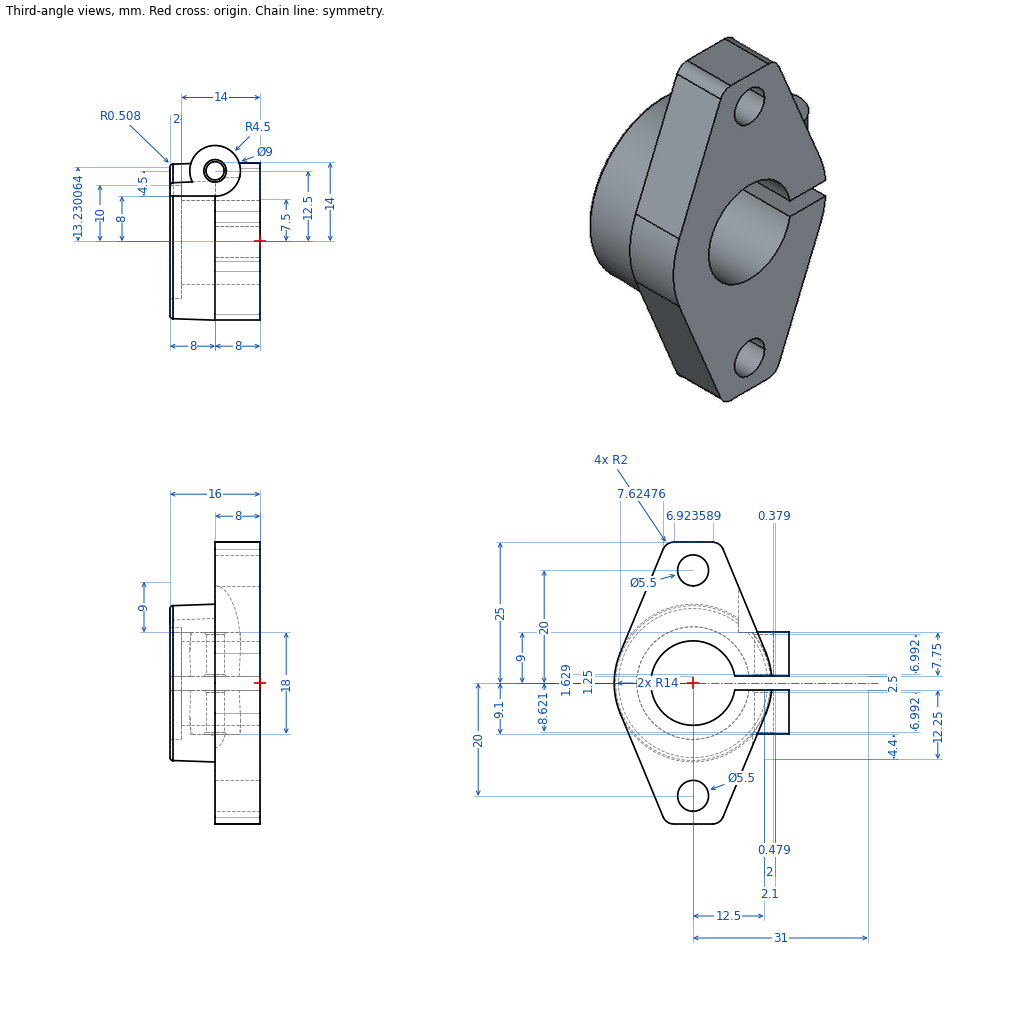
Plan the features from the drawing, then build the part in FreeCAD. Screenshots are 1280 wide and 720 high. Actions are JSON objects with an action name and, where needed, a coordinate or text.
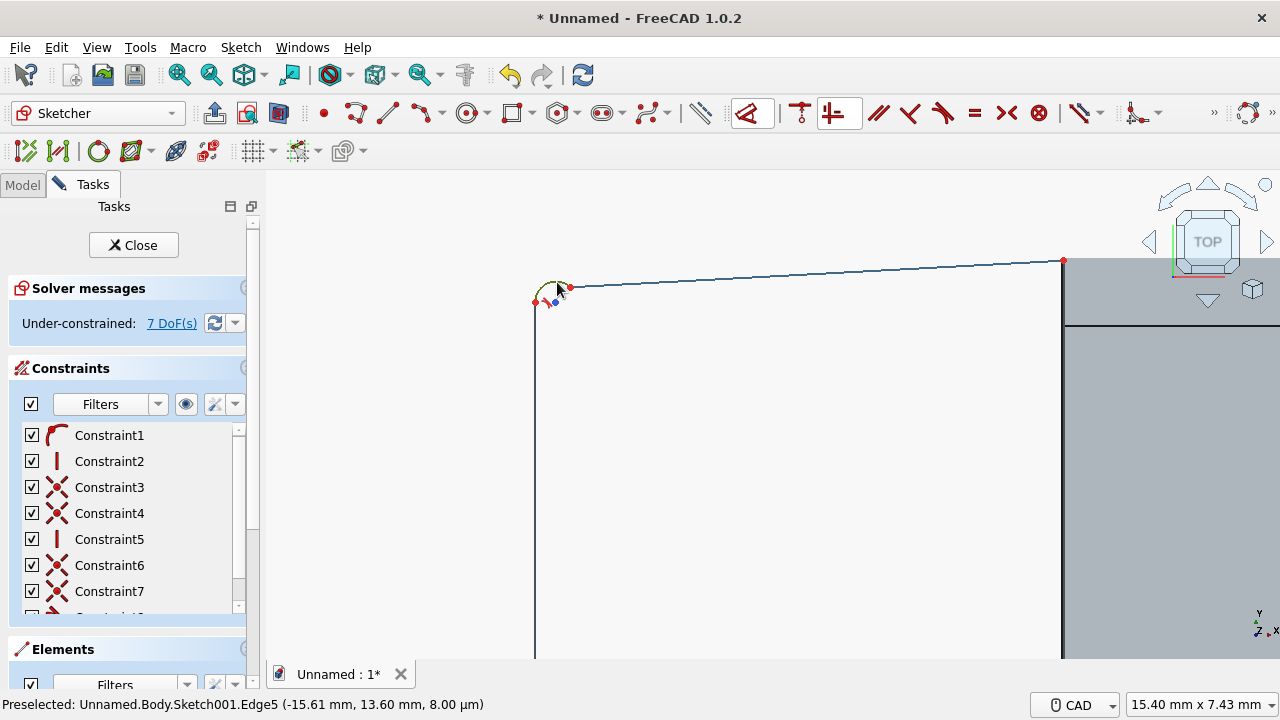
{"action": "left_click", "coordinate": [944, 114]}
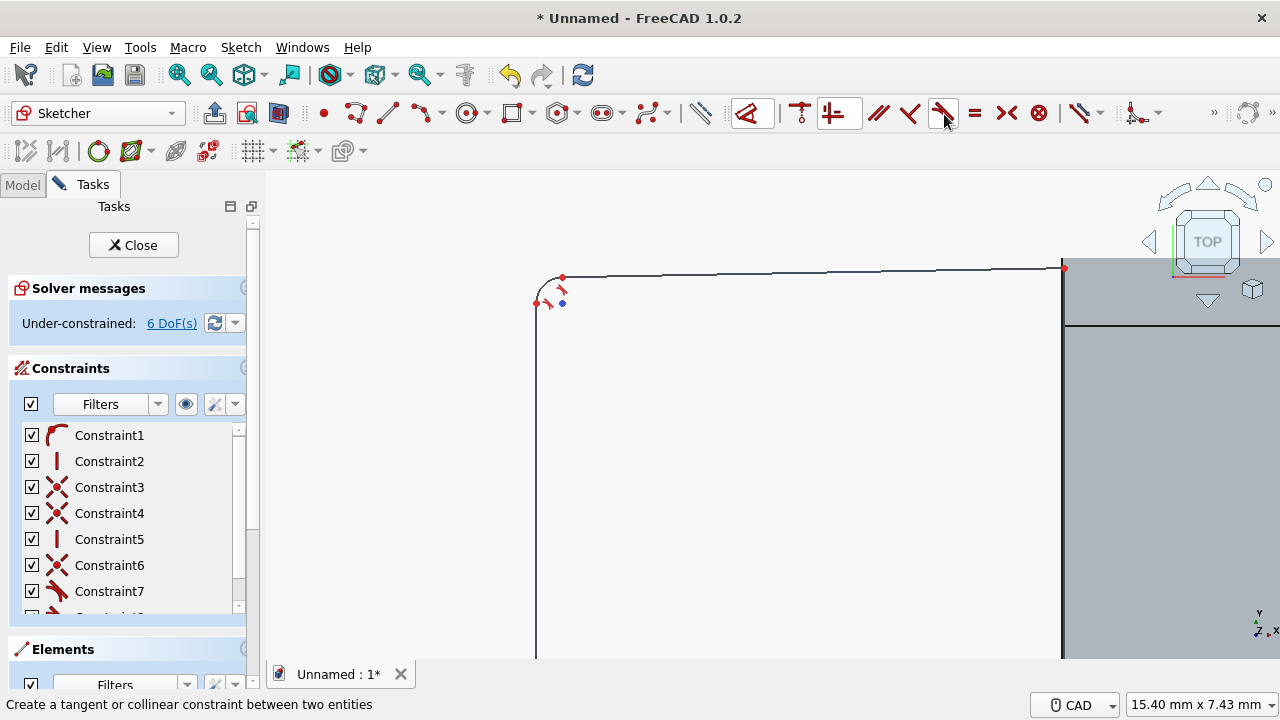
{"action": "scroll", "coordinate": [550, 284], "scroll_direction": "down", "scroll_amount": 6}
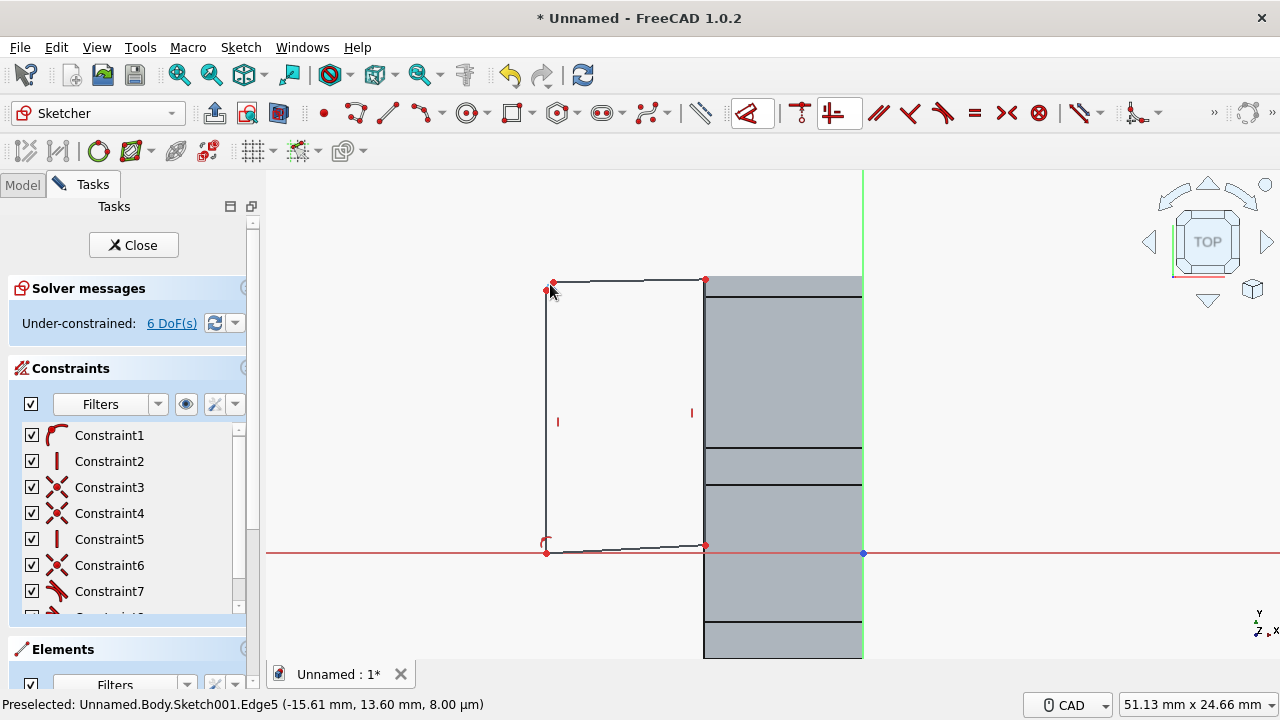
{"action": "scroll", "coordinate": [657, 548], "scroll_direction": "up", "scroll_amount": 5}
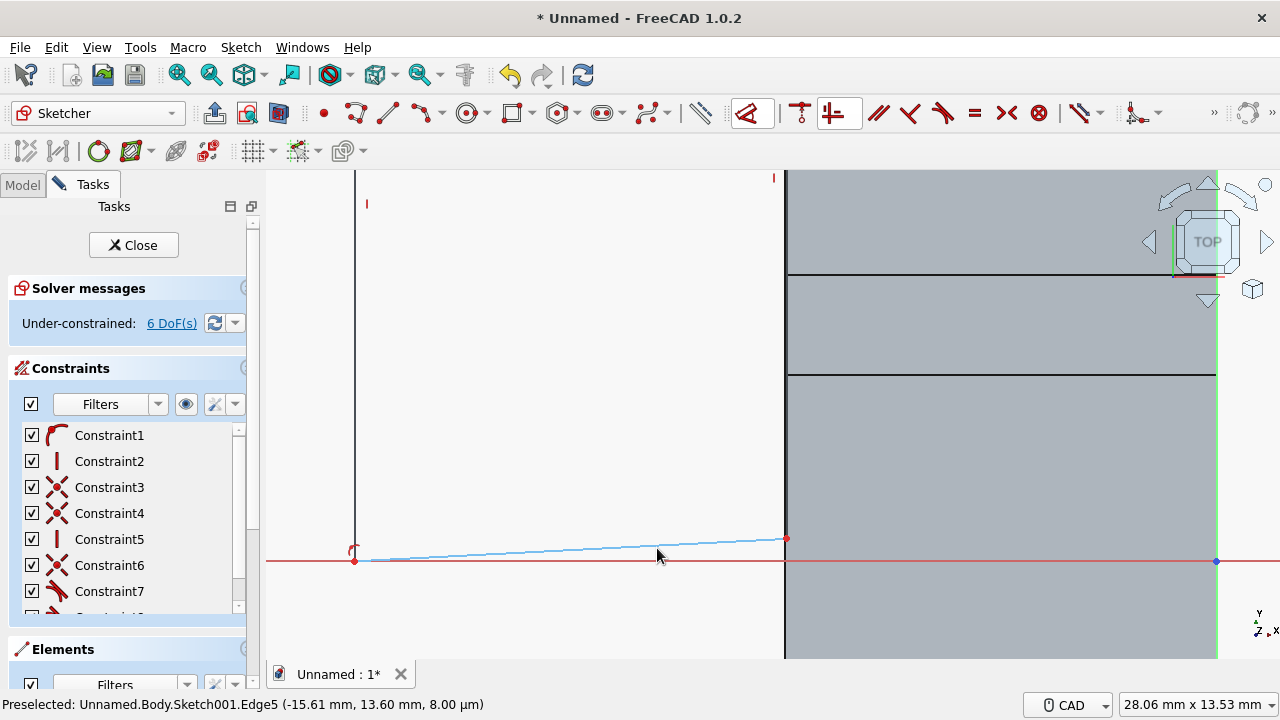
{"action": "left_click", "coordinate": [657, 546]}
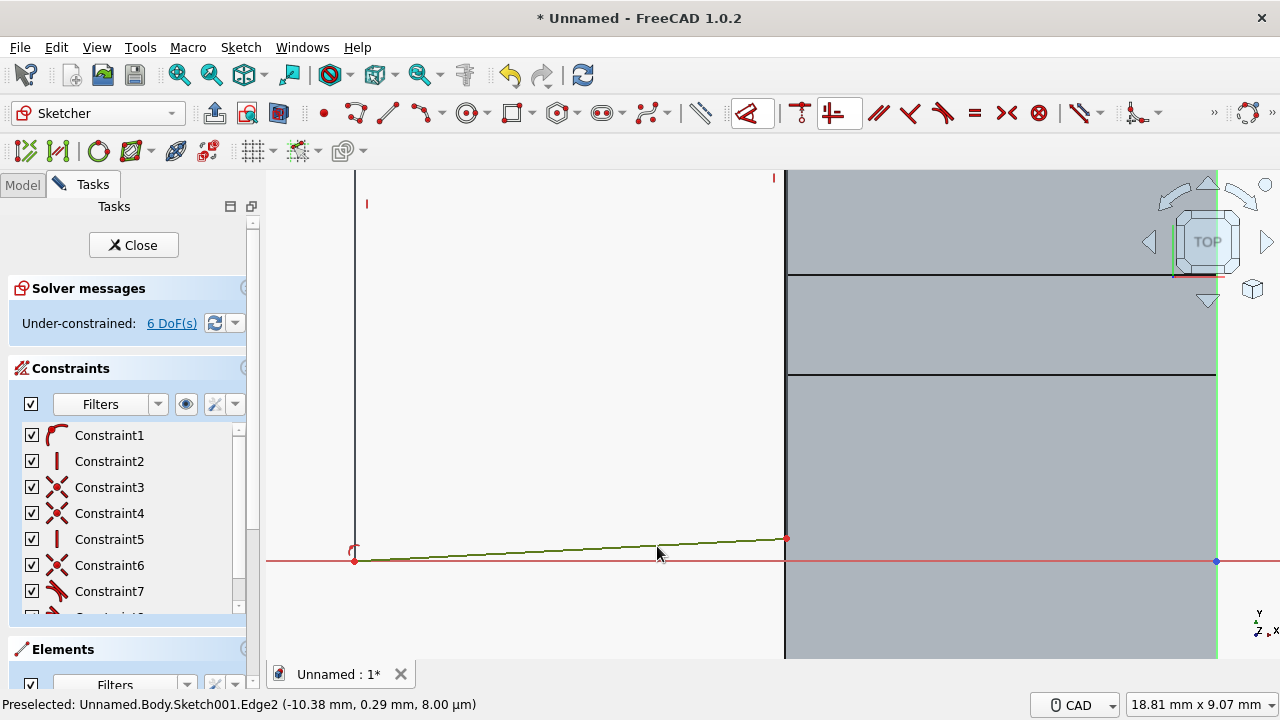
{"action": "key", "text": "h"}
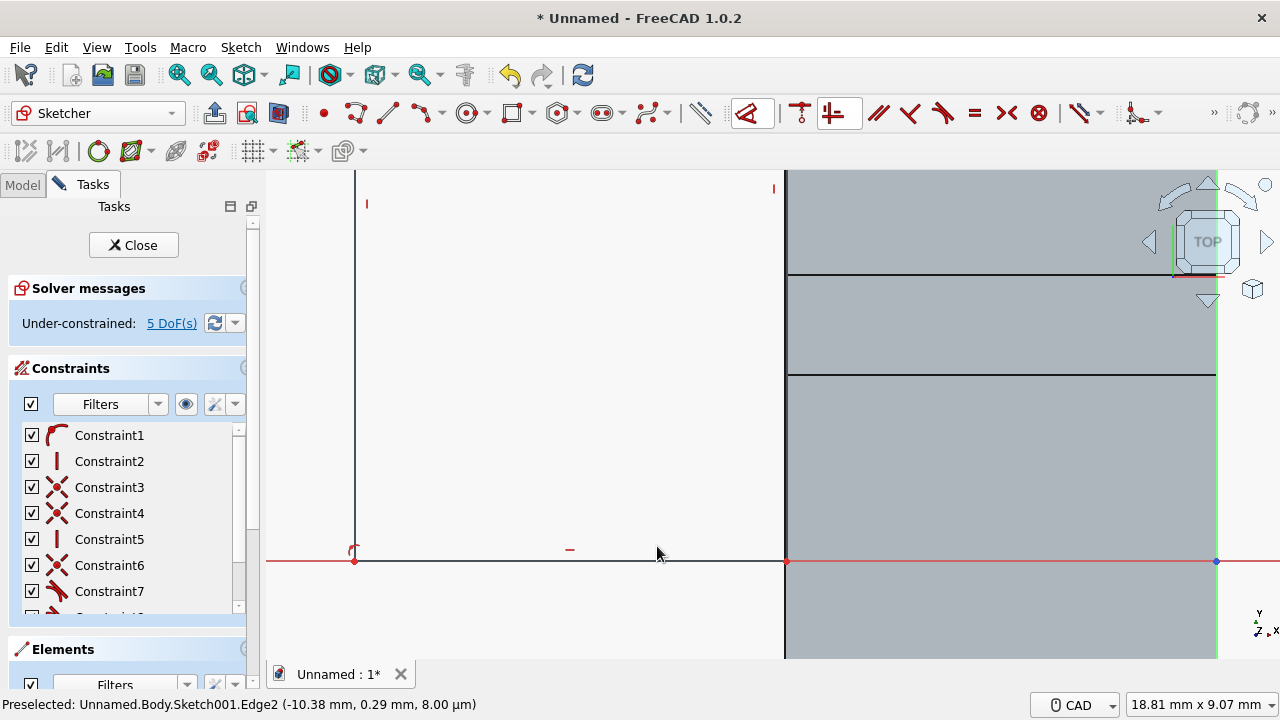
{"action": "scroll", "coordinate": [657, 549], "scroll_direction": "down", "scroll_amount": 5}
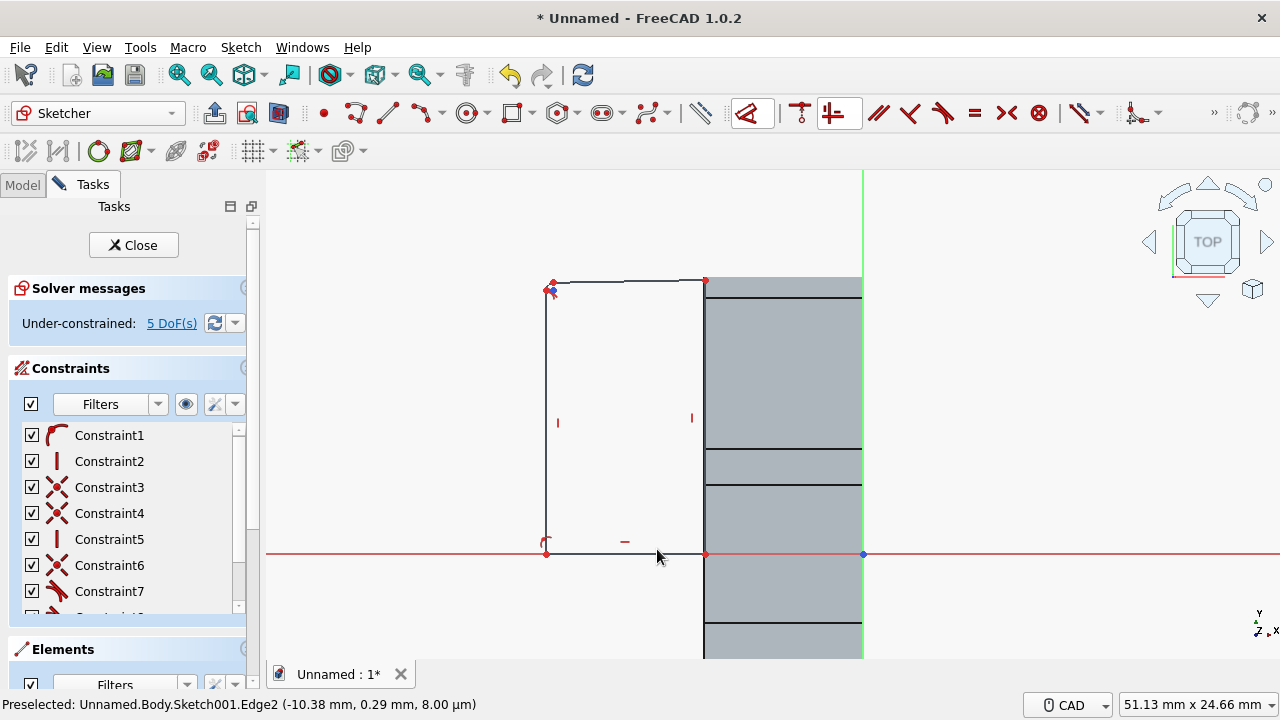
{"action": "scroll", "coordinate": [550, 284], "scroll_direction": "up", "scroll_amount": 7}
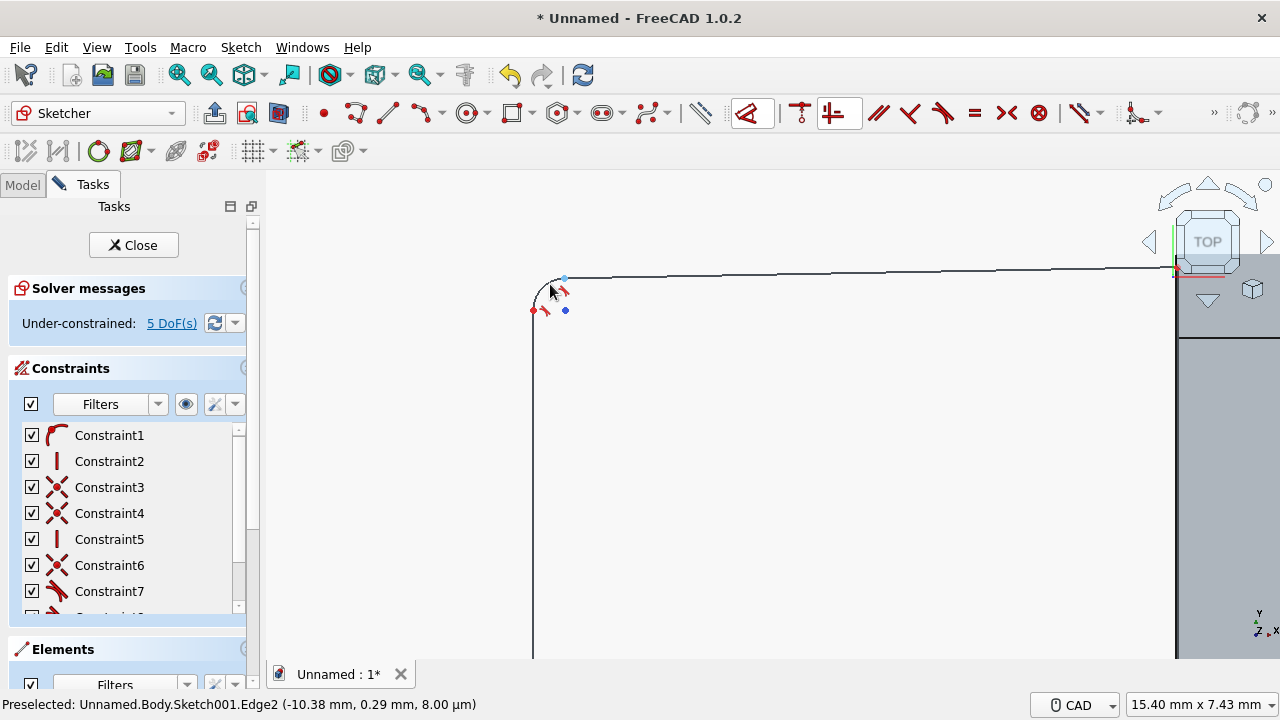
{"action": "left_click", "coordinate": [550, 282]}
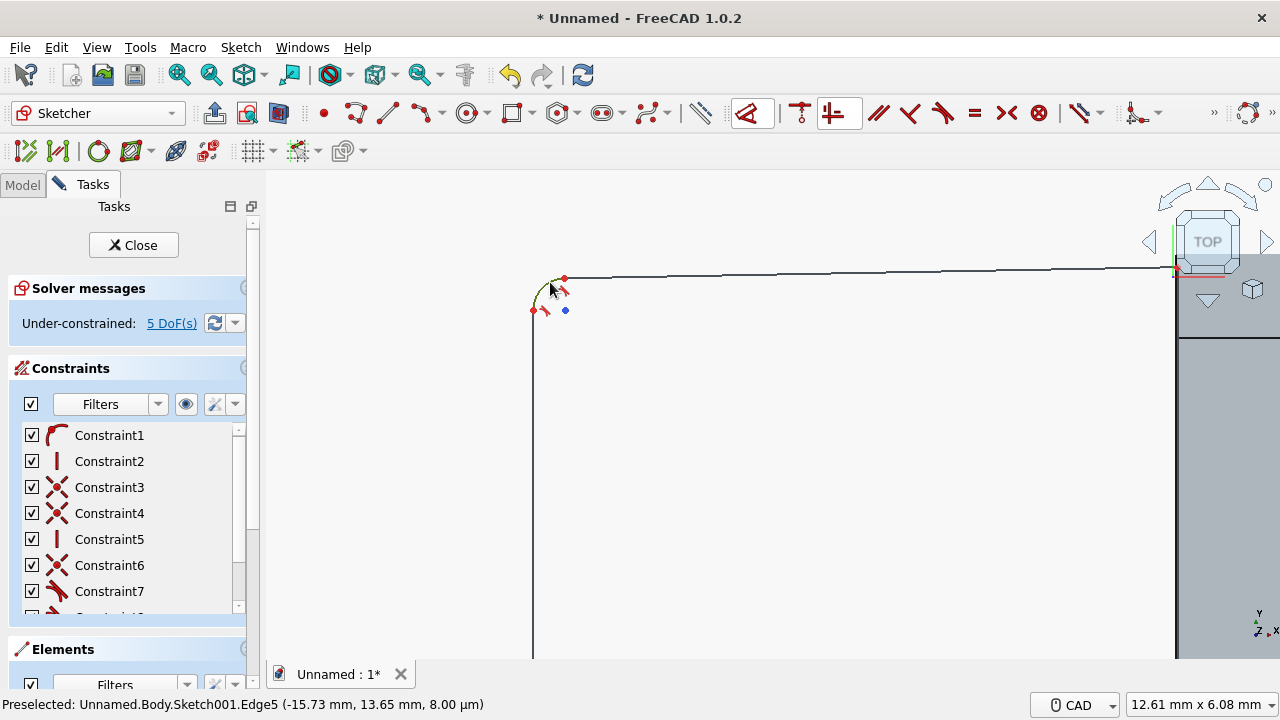
{"action": "key", "text": "k r"}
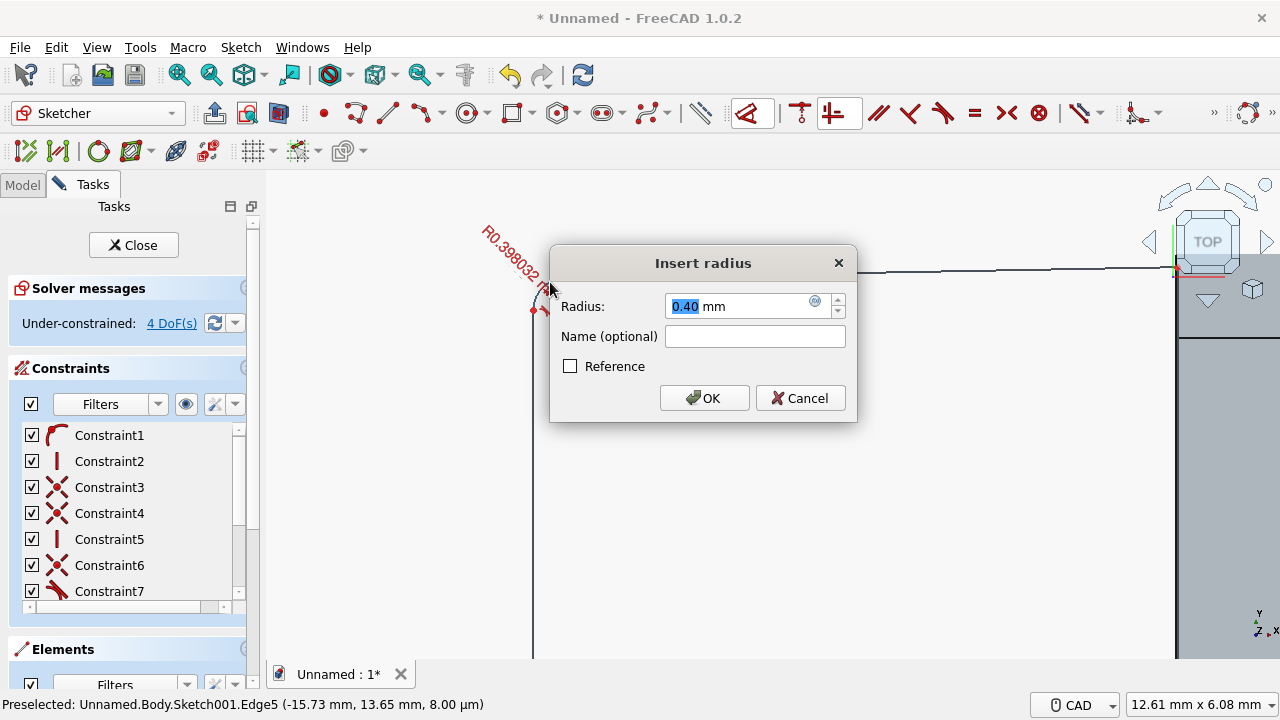
{"action": "type", "text": "0.508"}
{"action": "key", "text": "Return"}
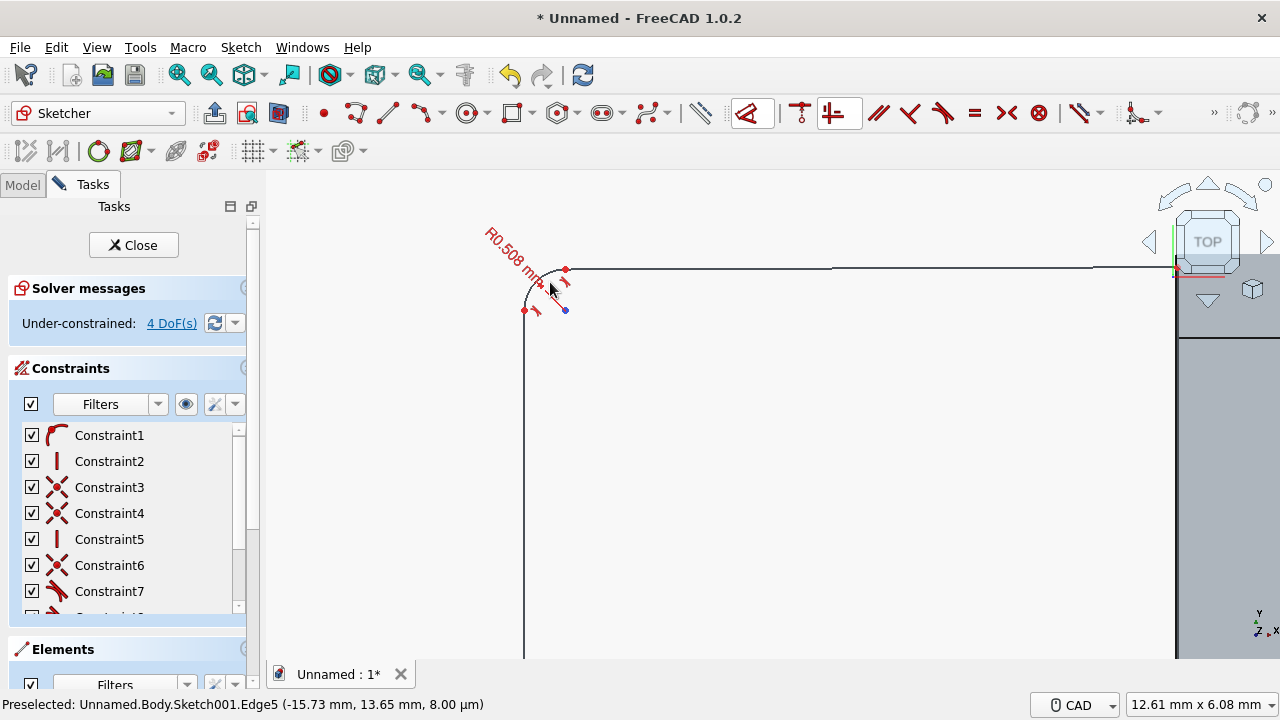
{"action": "scroll", "coordinate": [550, 283], "scroll_direction": "down", "scroll_amount": 7}